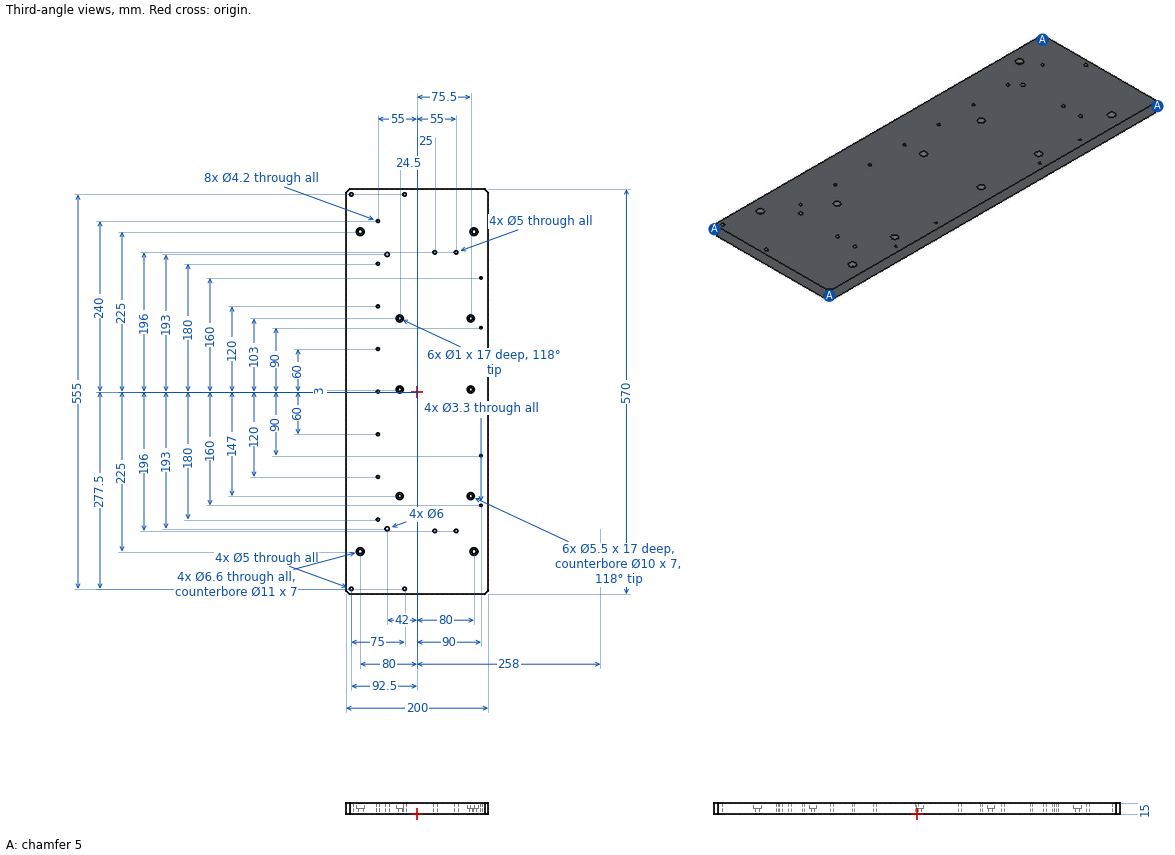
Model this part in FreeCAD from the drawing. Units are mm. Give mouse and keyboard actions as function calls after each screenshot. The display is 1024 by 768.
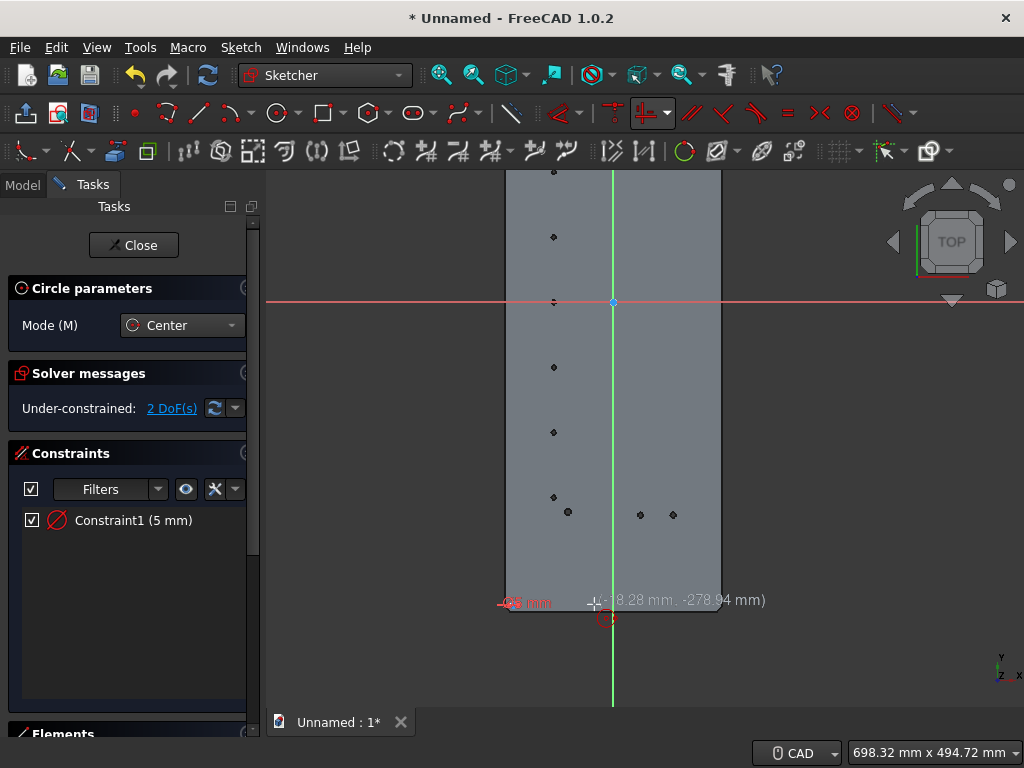
click(594, 604)
move(596, 602)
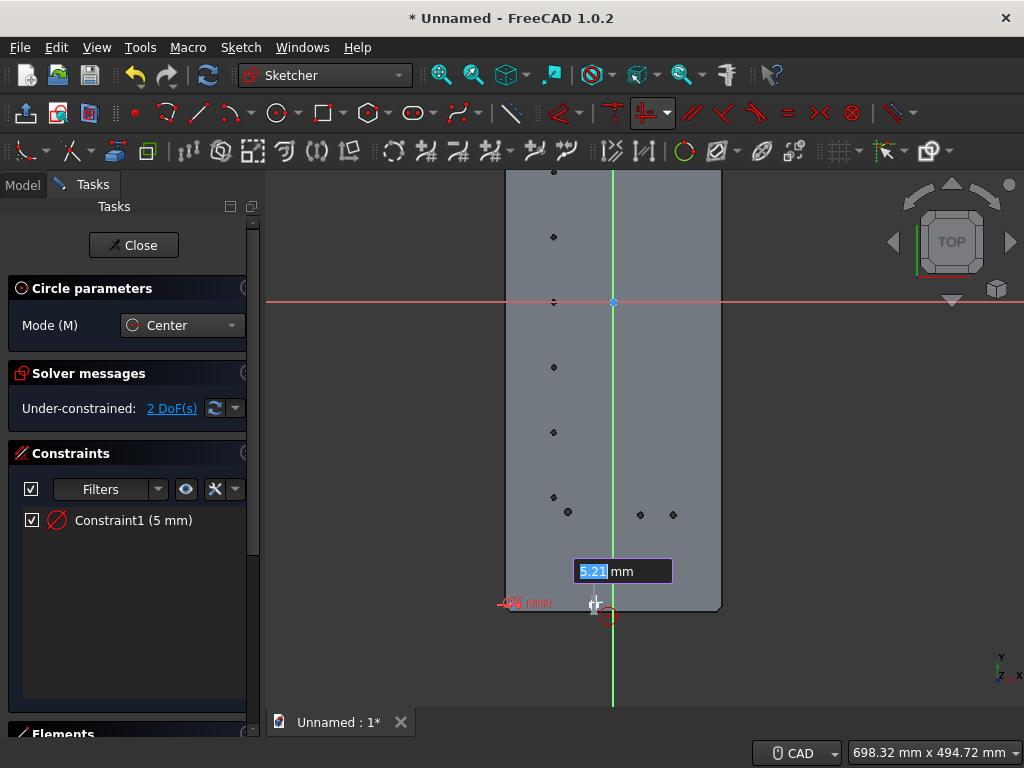
text(5)
key(Return)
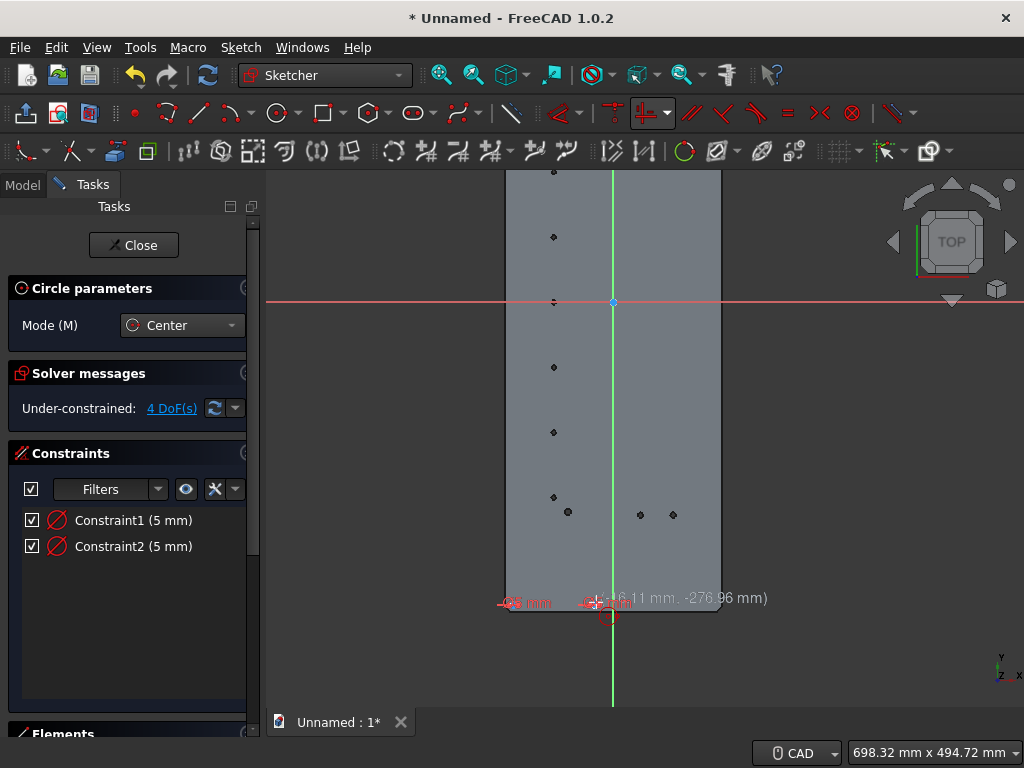
scroll(594, 604, down, 3)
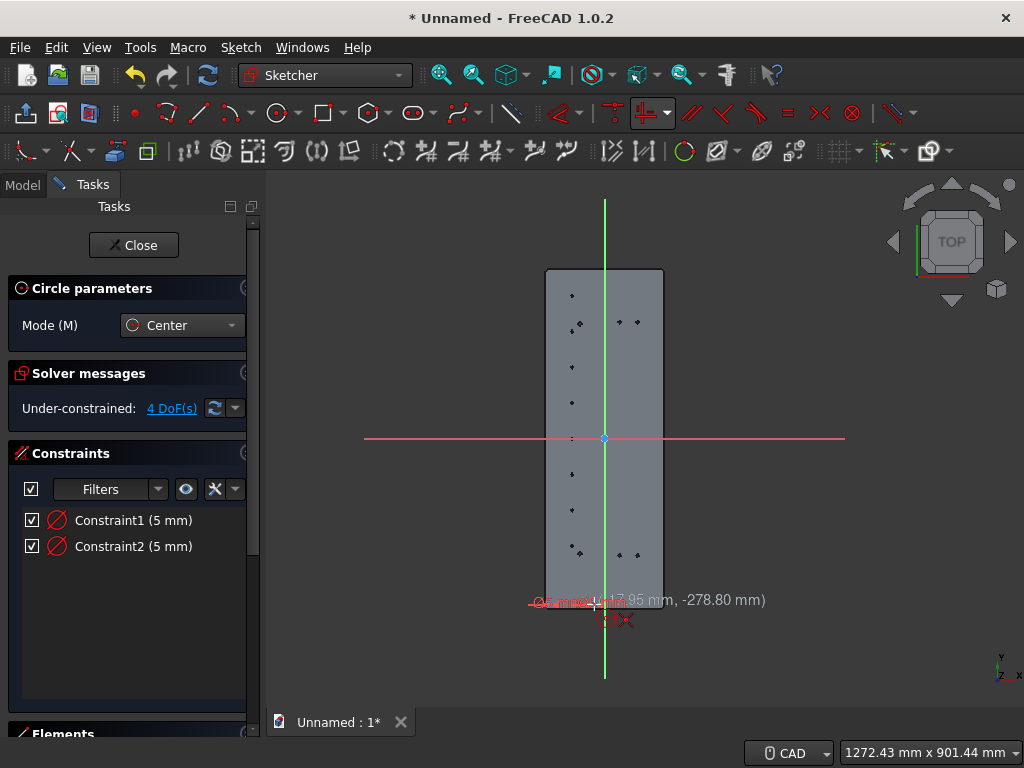
scroll(594, 274, up, 14)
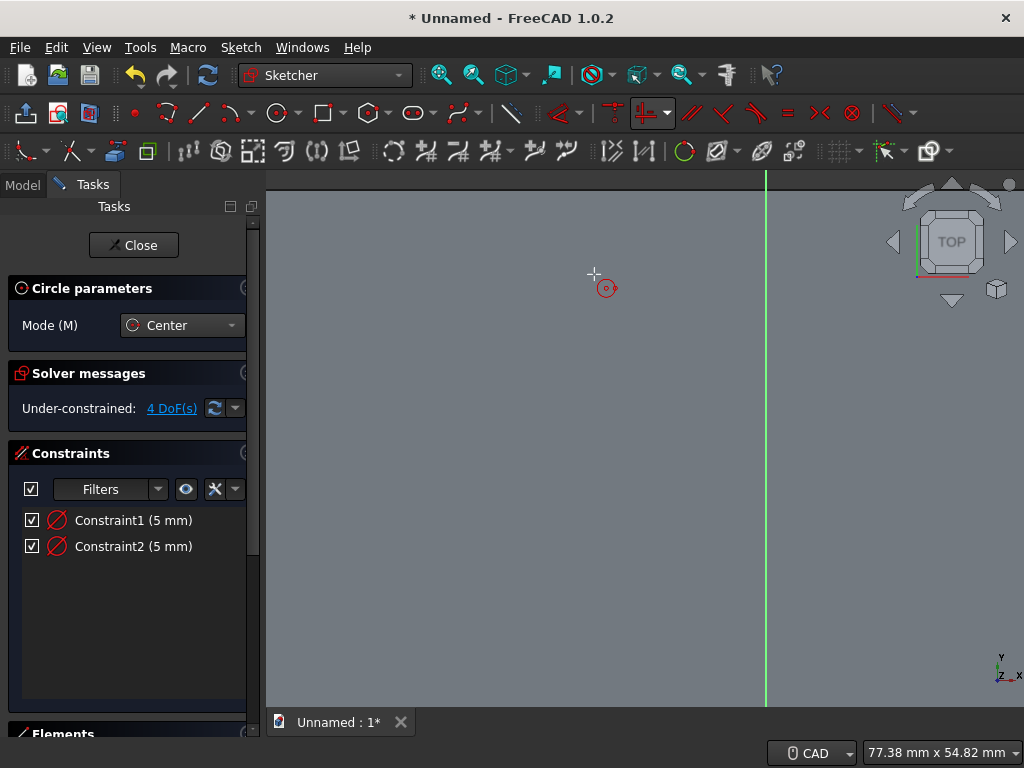
scroll(594, 274, down, 14)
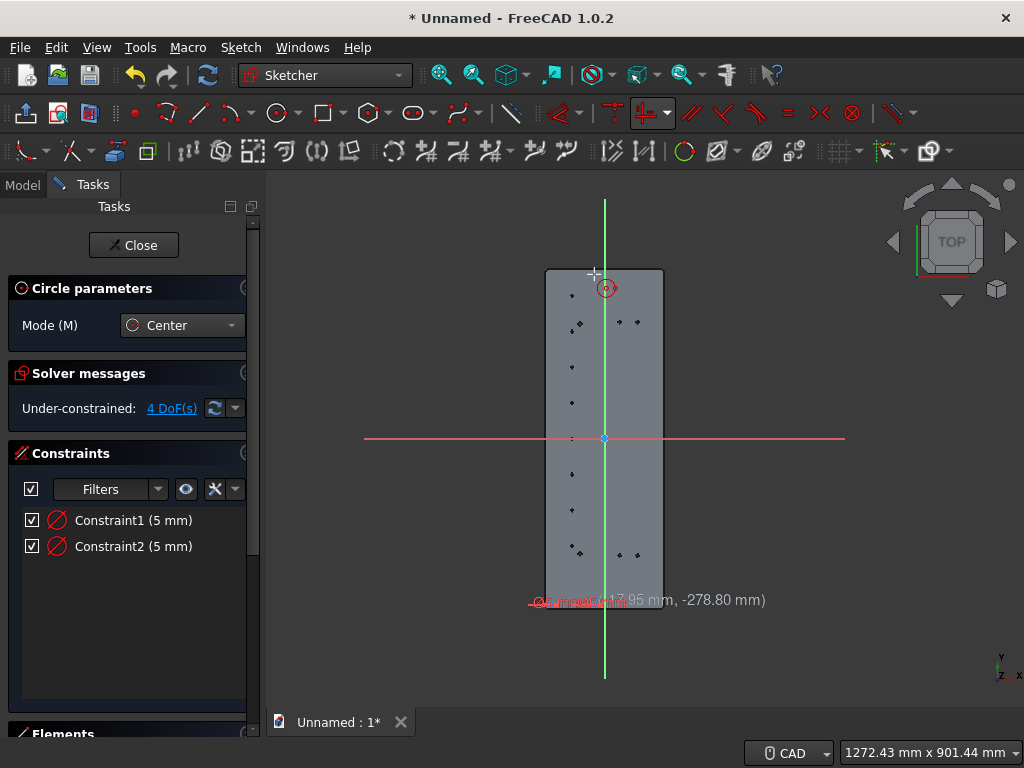
scroll(594, 274, up, 3)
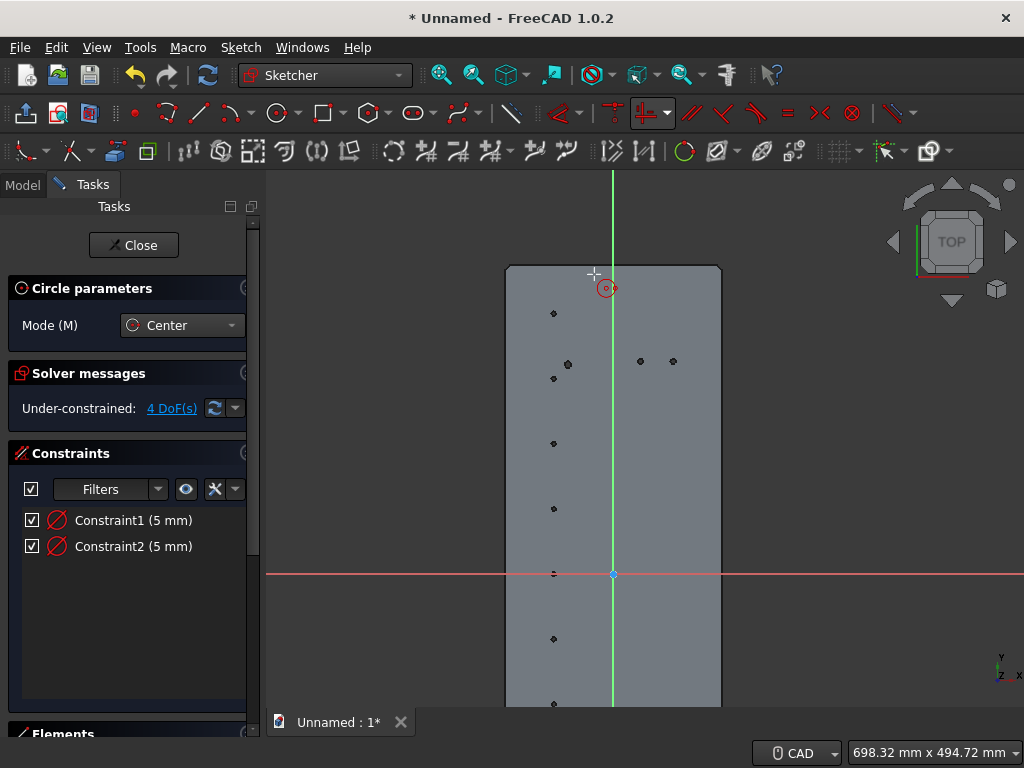
click(594, 273)
move(596, 271)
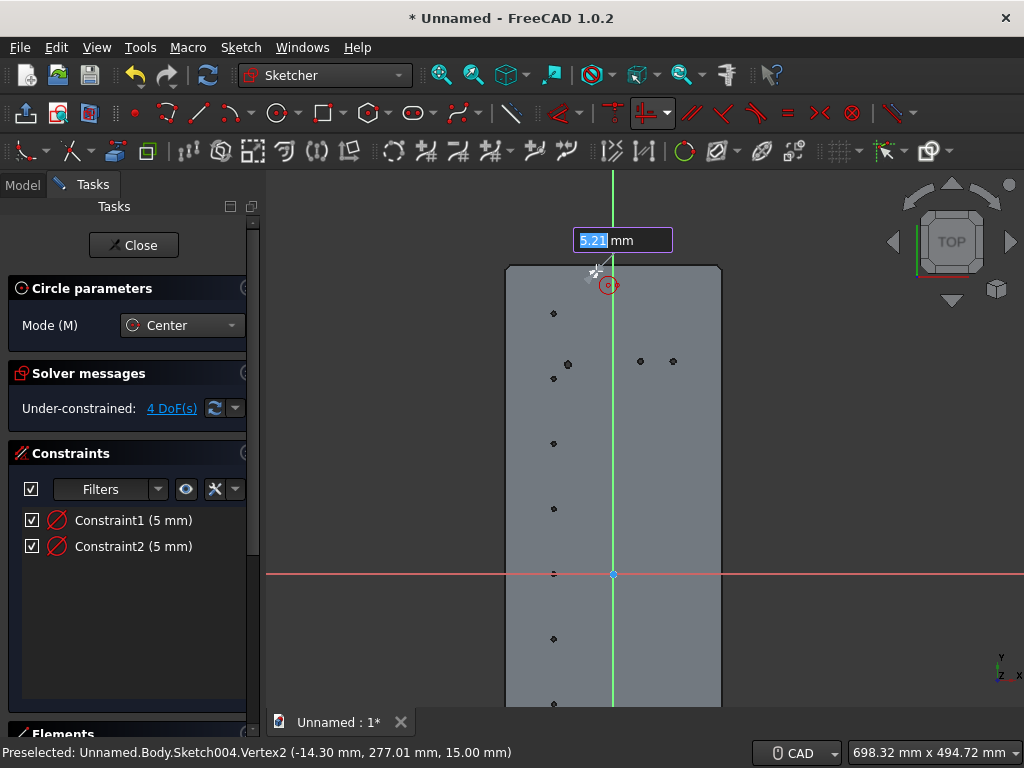
text(5)
key(Return)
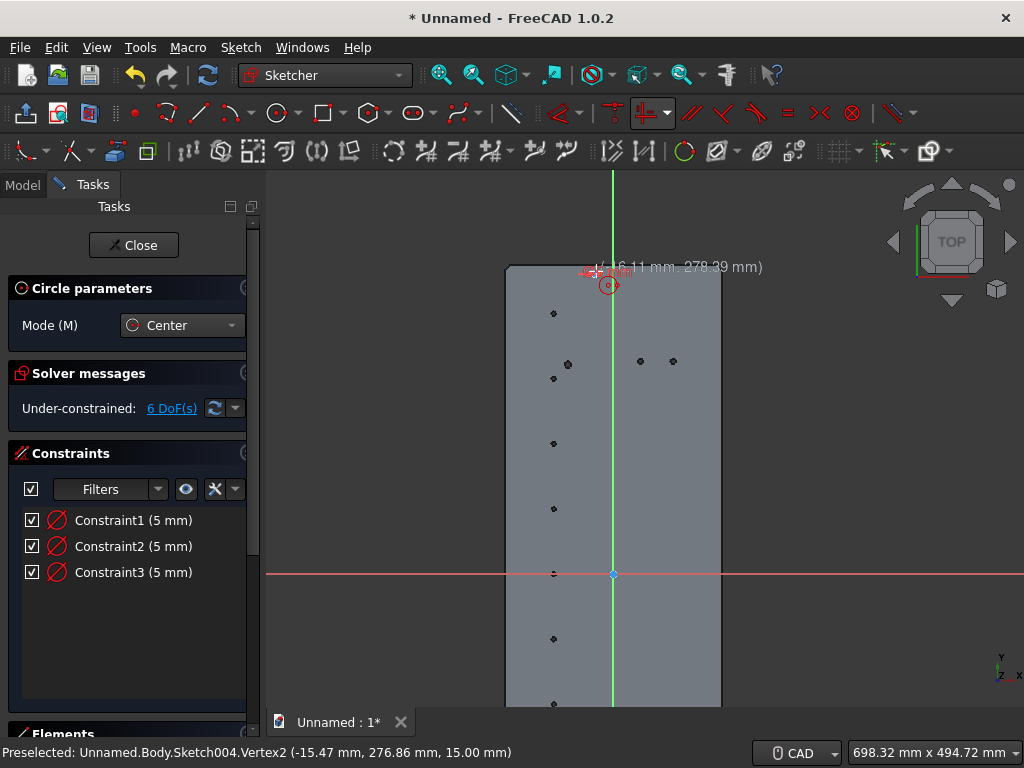
scroll(513, 273, up, 11)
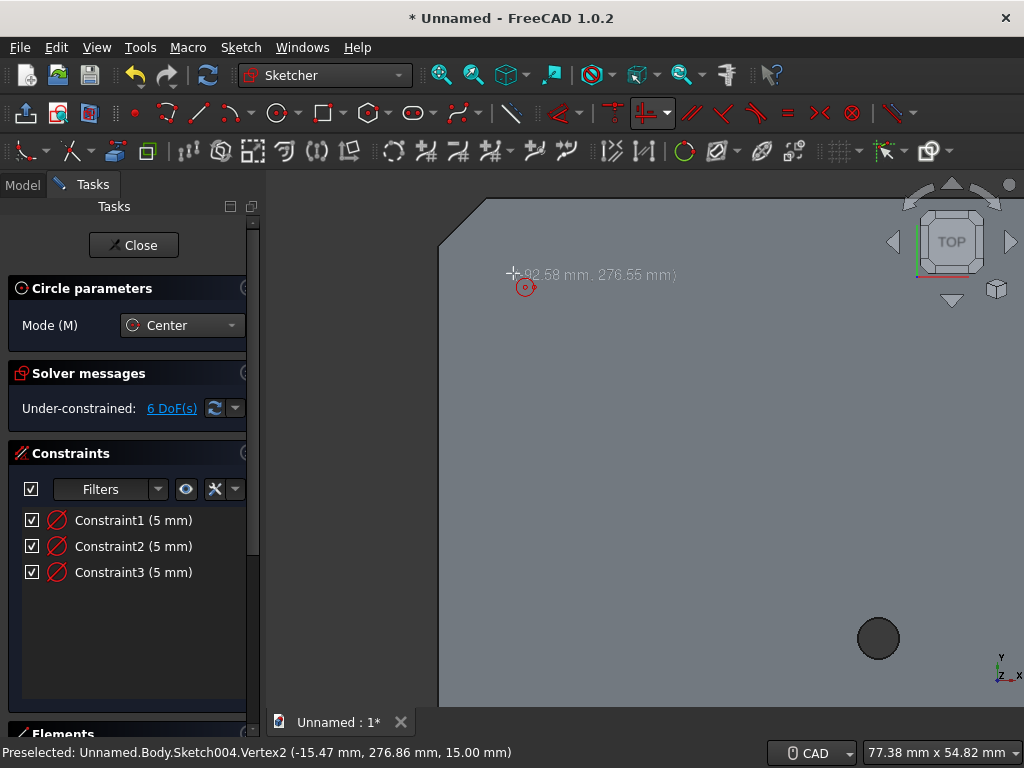
scroll(552, 273, down, 14)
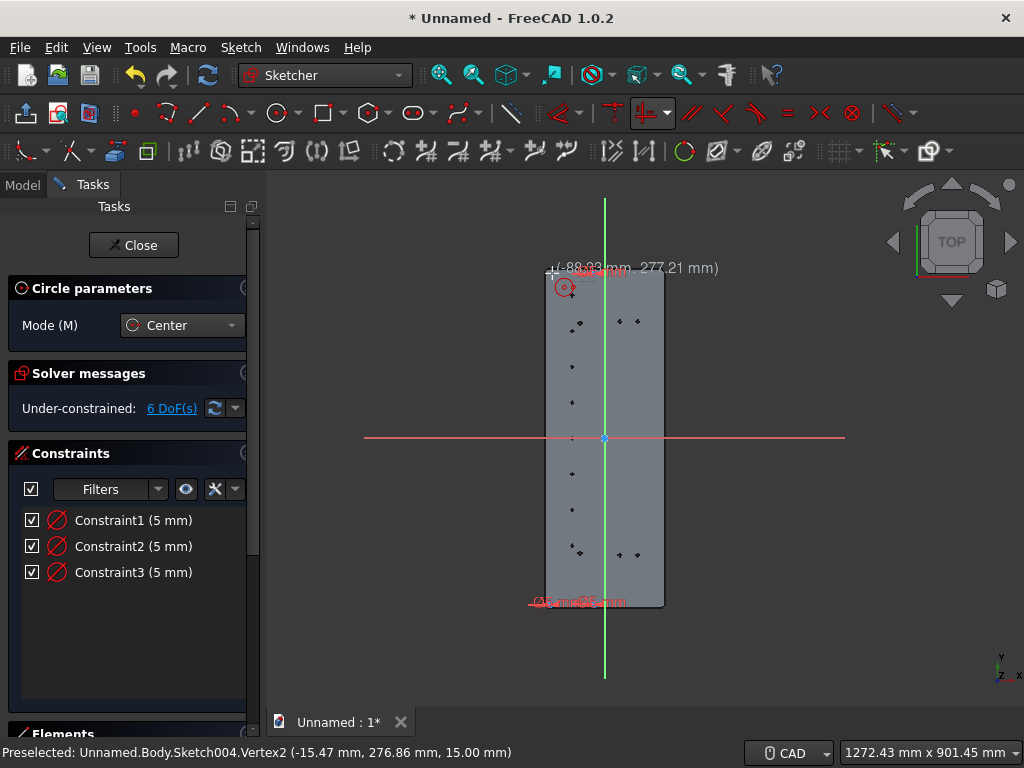
click(550, 273)
move(551, 272)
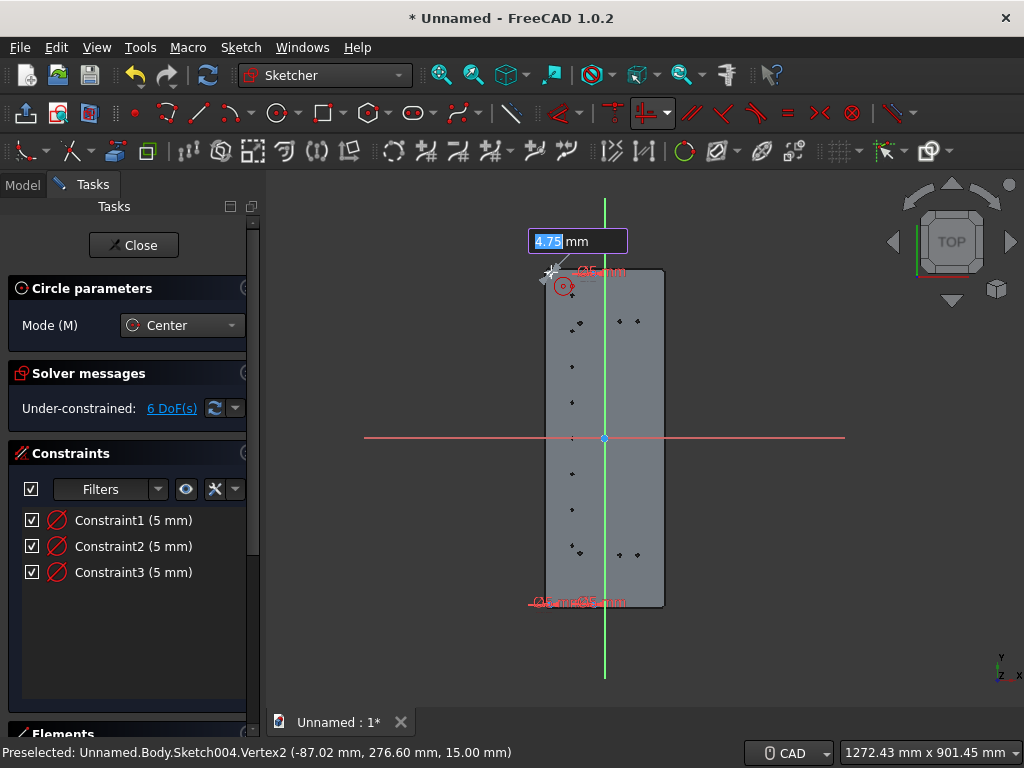
text(5)
key(Return)
key(Escape)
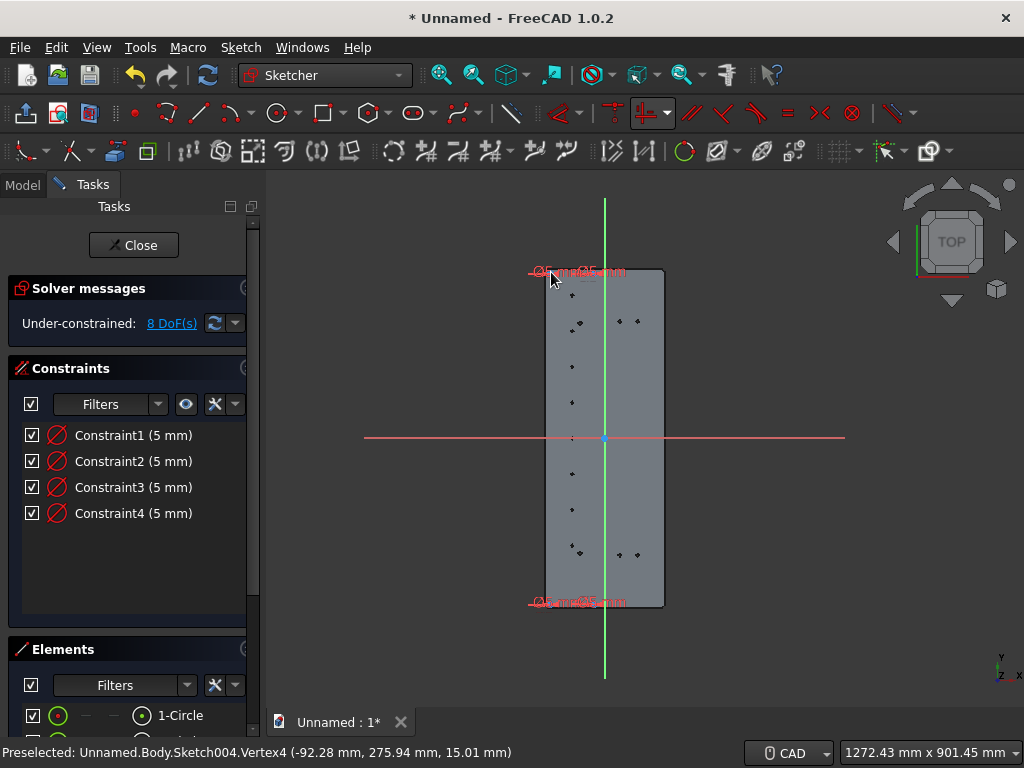
click(550, 605)